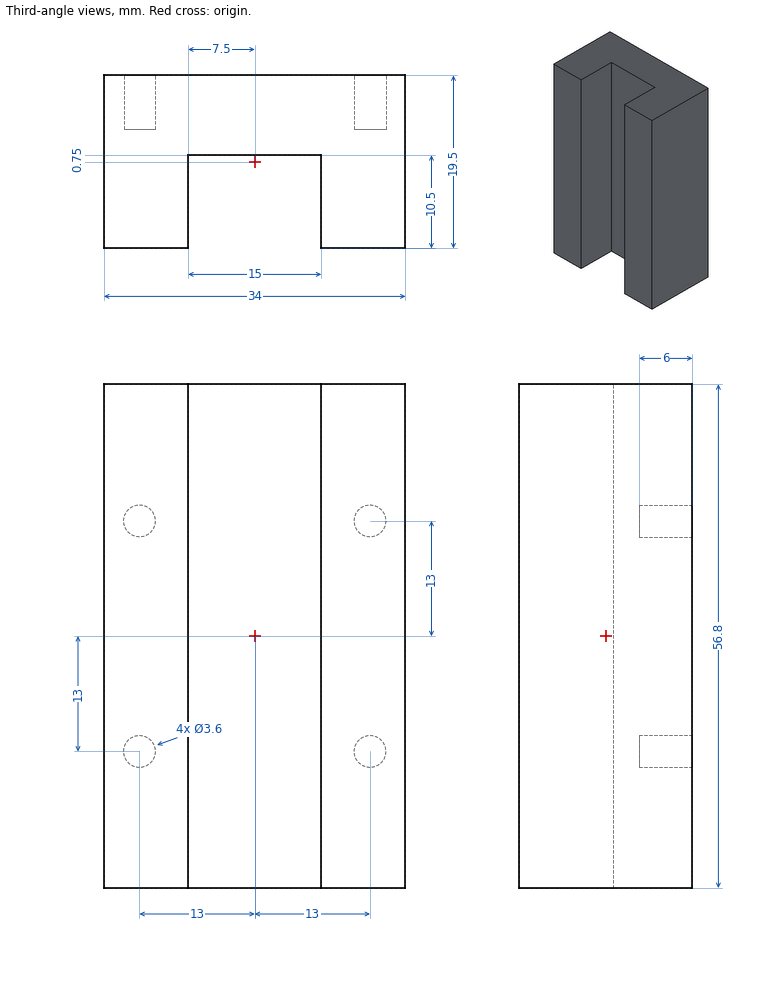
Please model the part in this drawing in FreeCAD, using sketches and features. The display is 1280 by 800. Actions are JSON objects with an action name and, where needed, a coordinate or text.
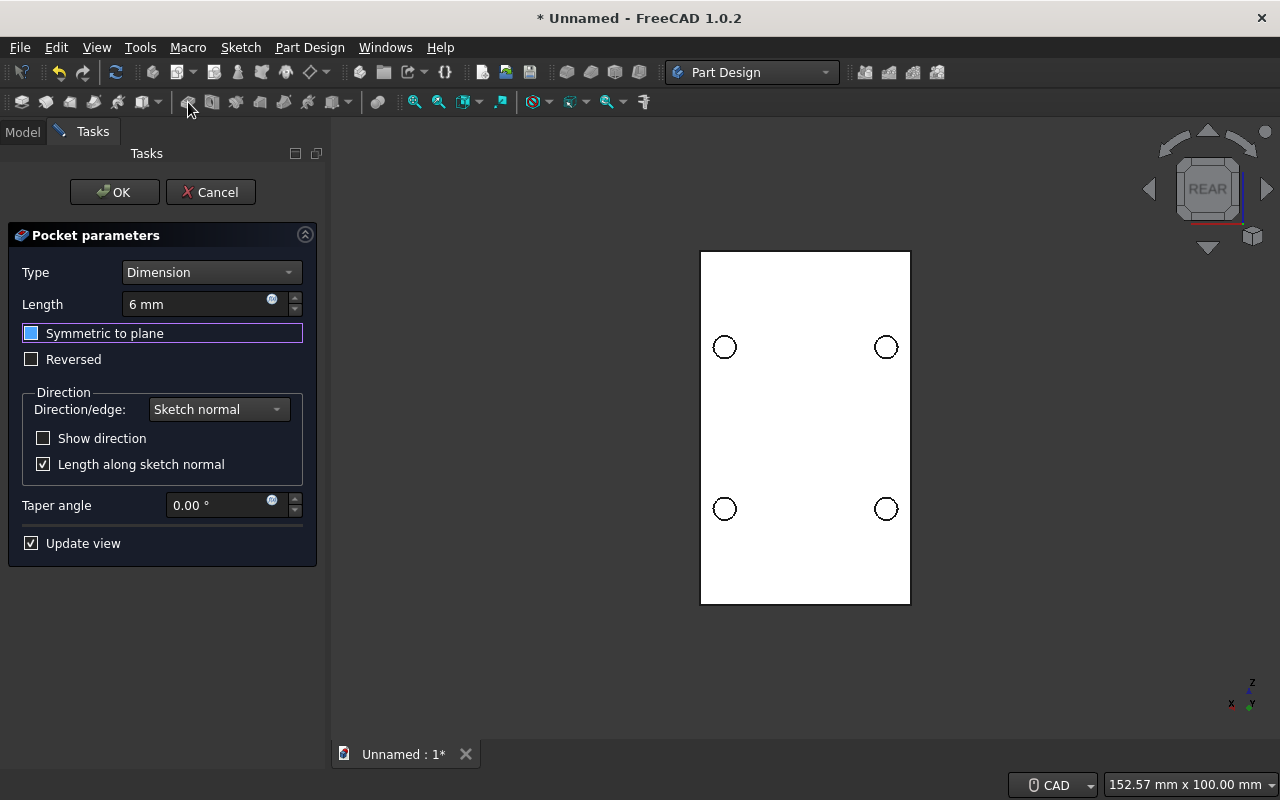
{"action": "left_click", "coordinate": [115, 192]}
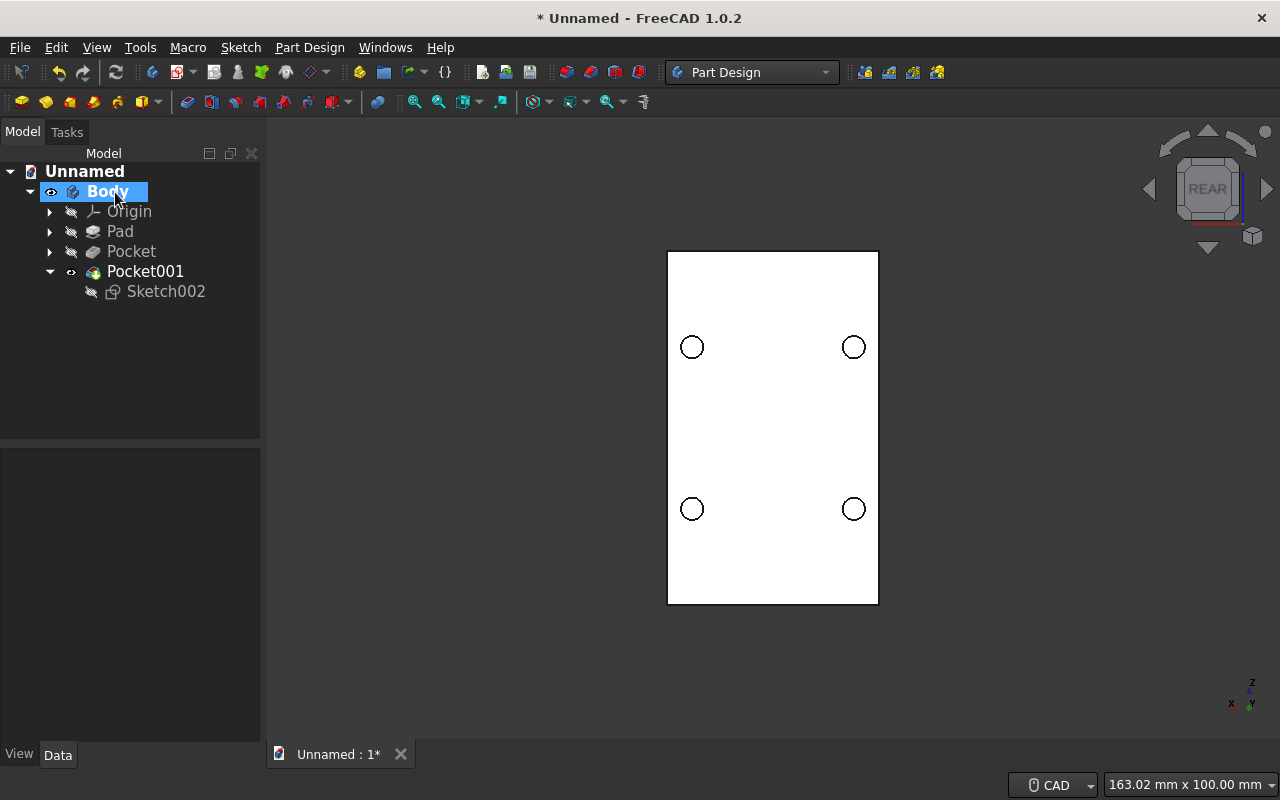
{"action": "key", "text": "0"}